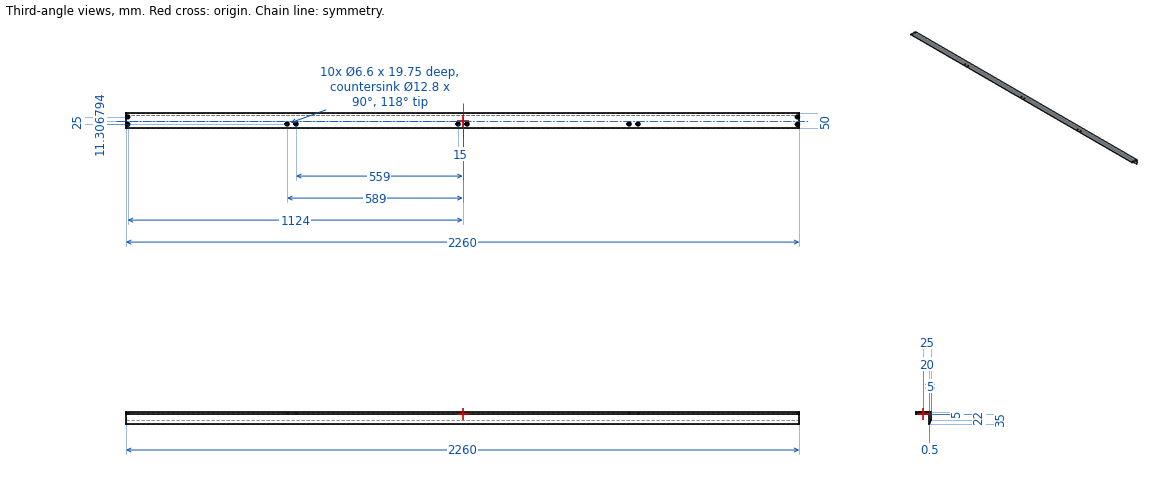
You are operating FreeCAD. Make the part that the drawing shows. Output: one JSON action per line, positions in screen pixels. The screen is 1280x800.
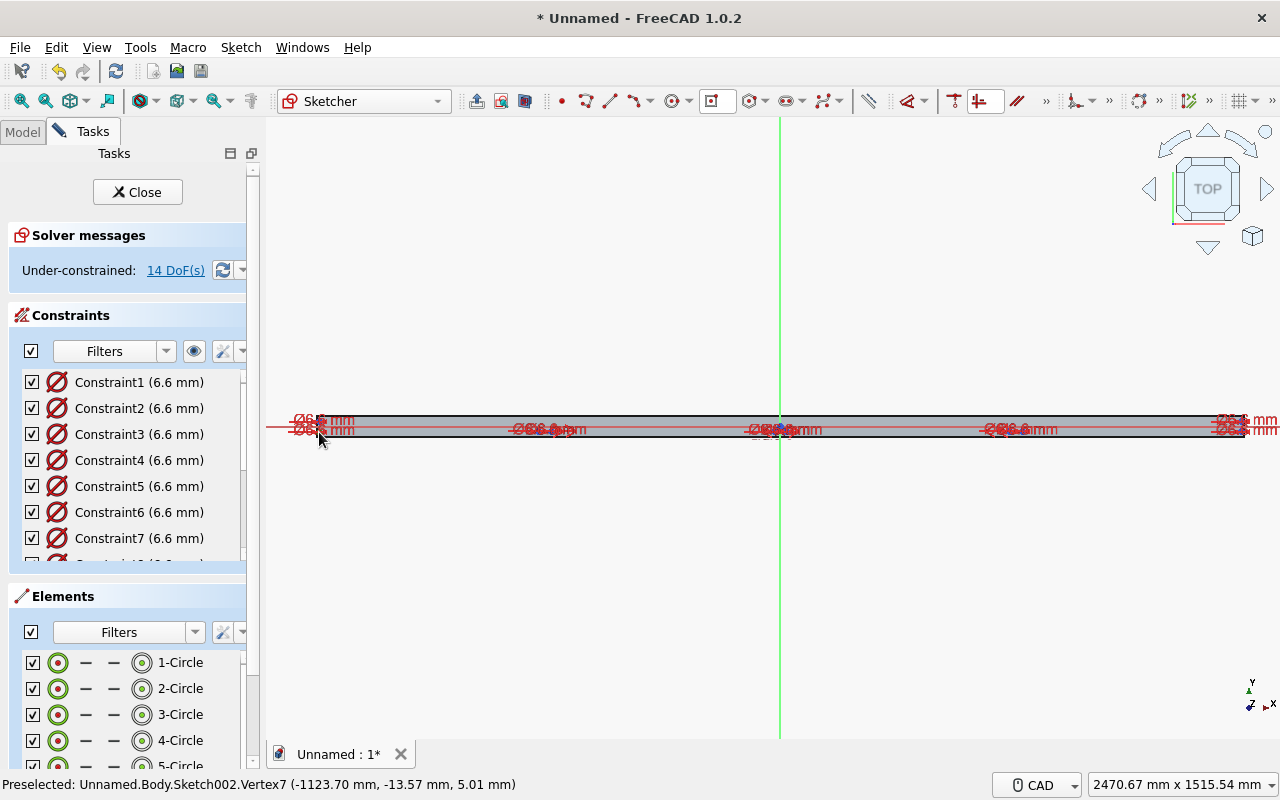
{"action": "left_click", "coordinate": [319, 422]}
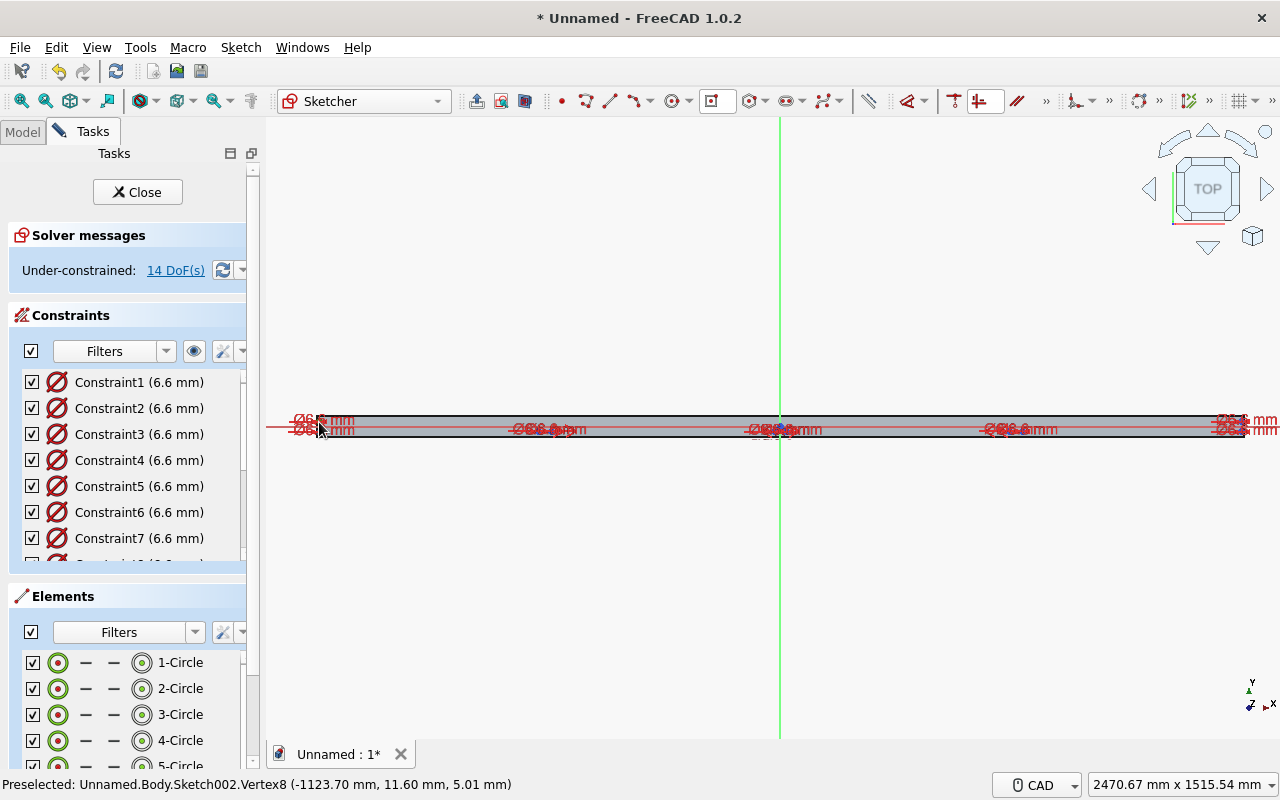
{"action": "left_click", "coordinate": [411, 427]}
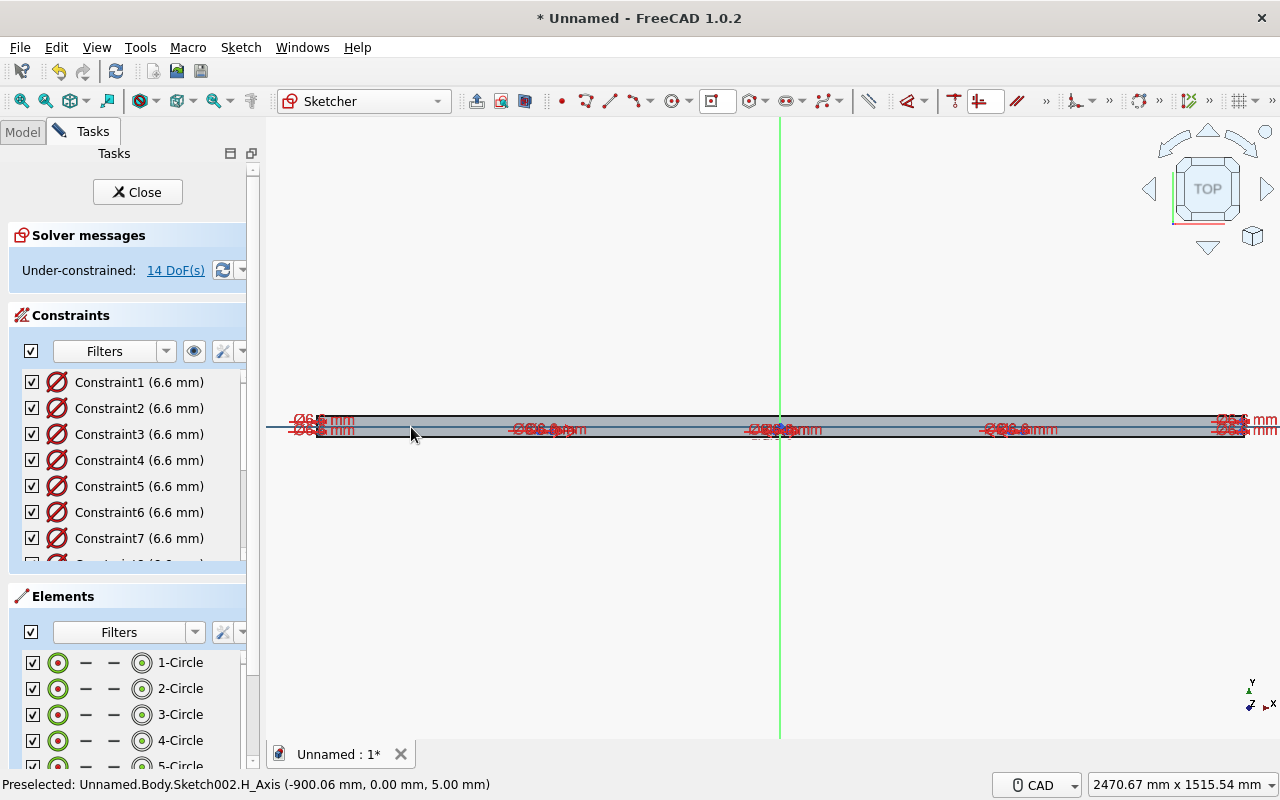
{"action": "key", "text": "s"}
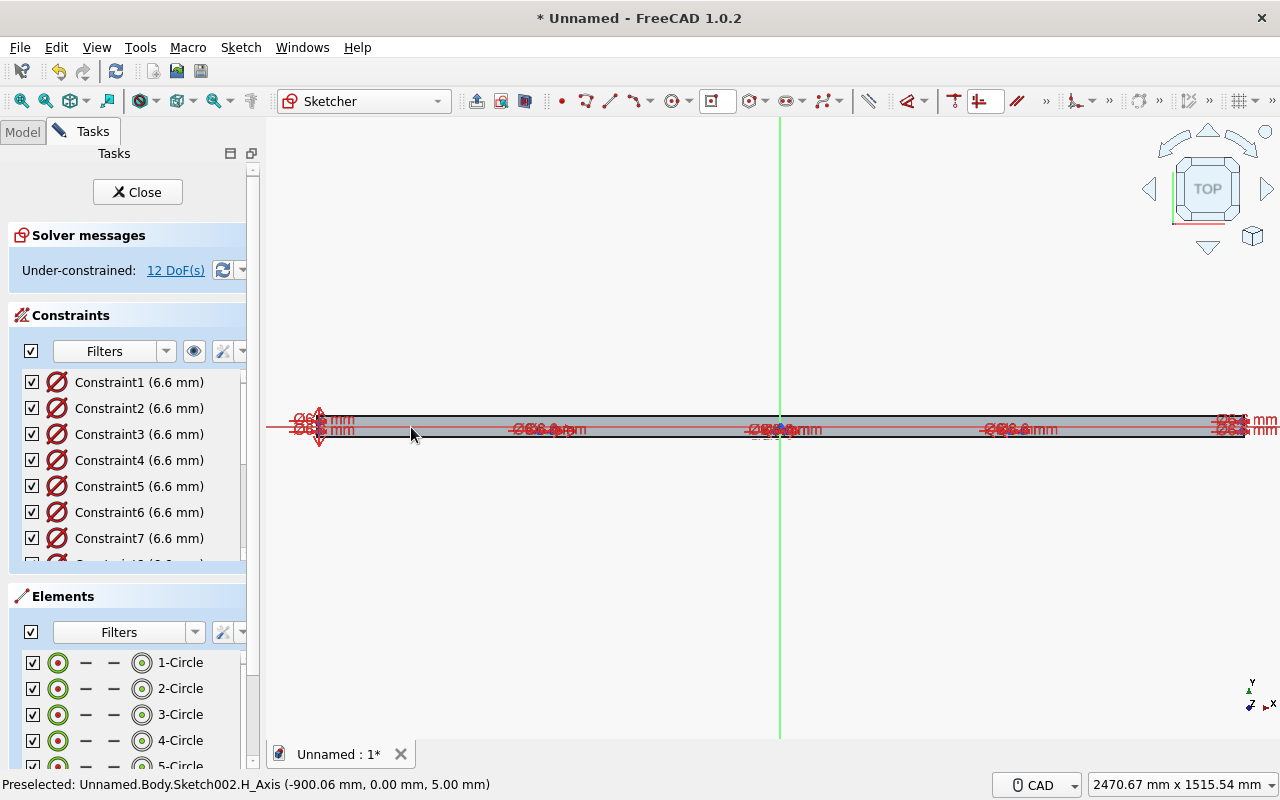
{"action": "left_click", "coordinate": [319, 432]}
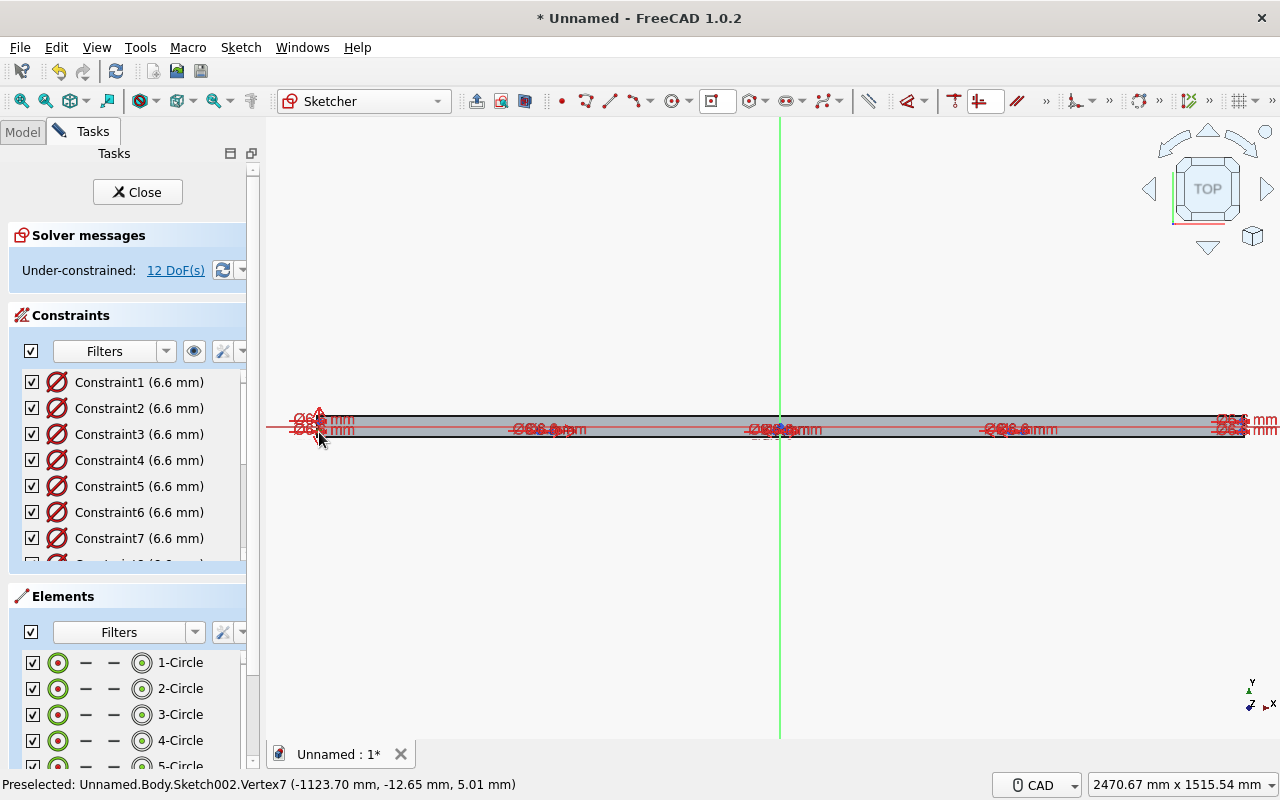
{"action": "scroll", "coordinate": [550, 431], "scroll_direction": "down", "scroll_amount": 2}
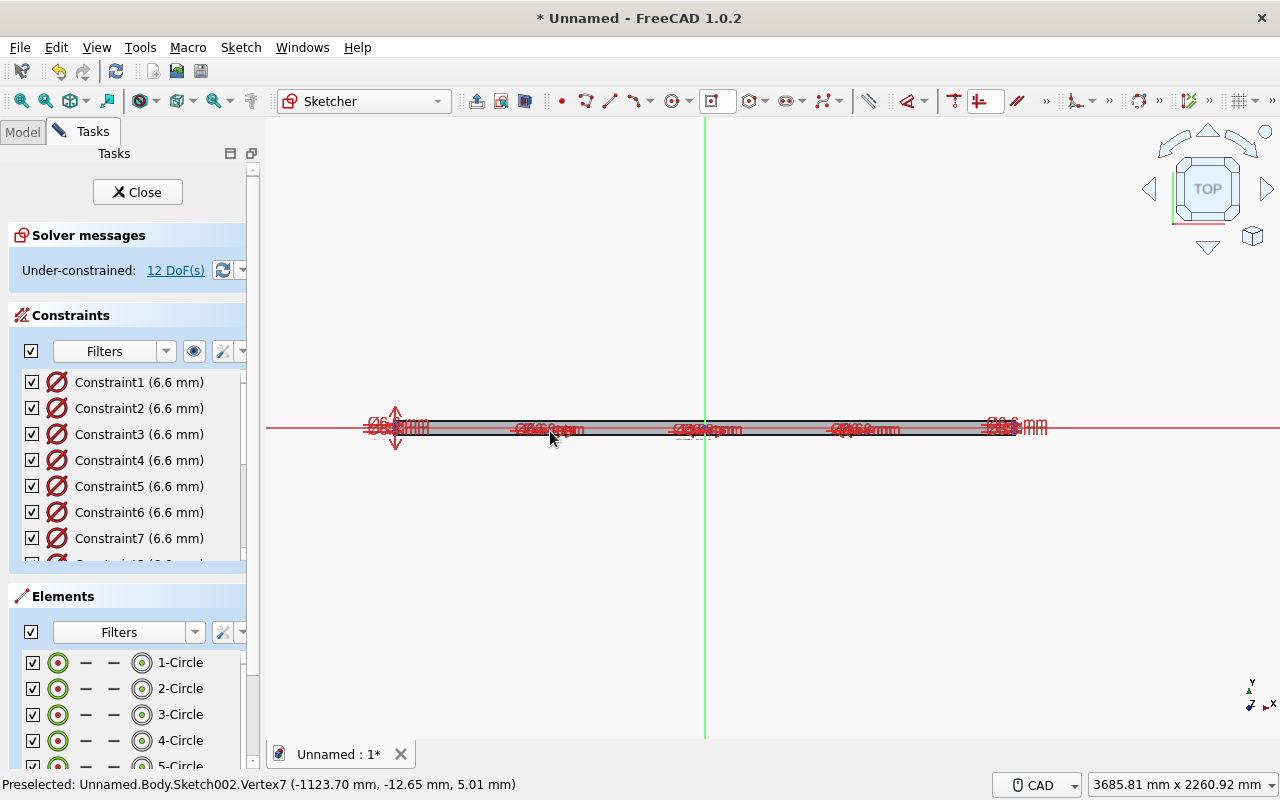
{"action": "scroll", "coordinate": [1014, 432], "scroll_direction": "up", "scroll_amount": 3}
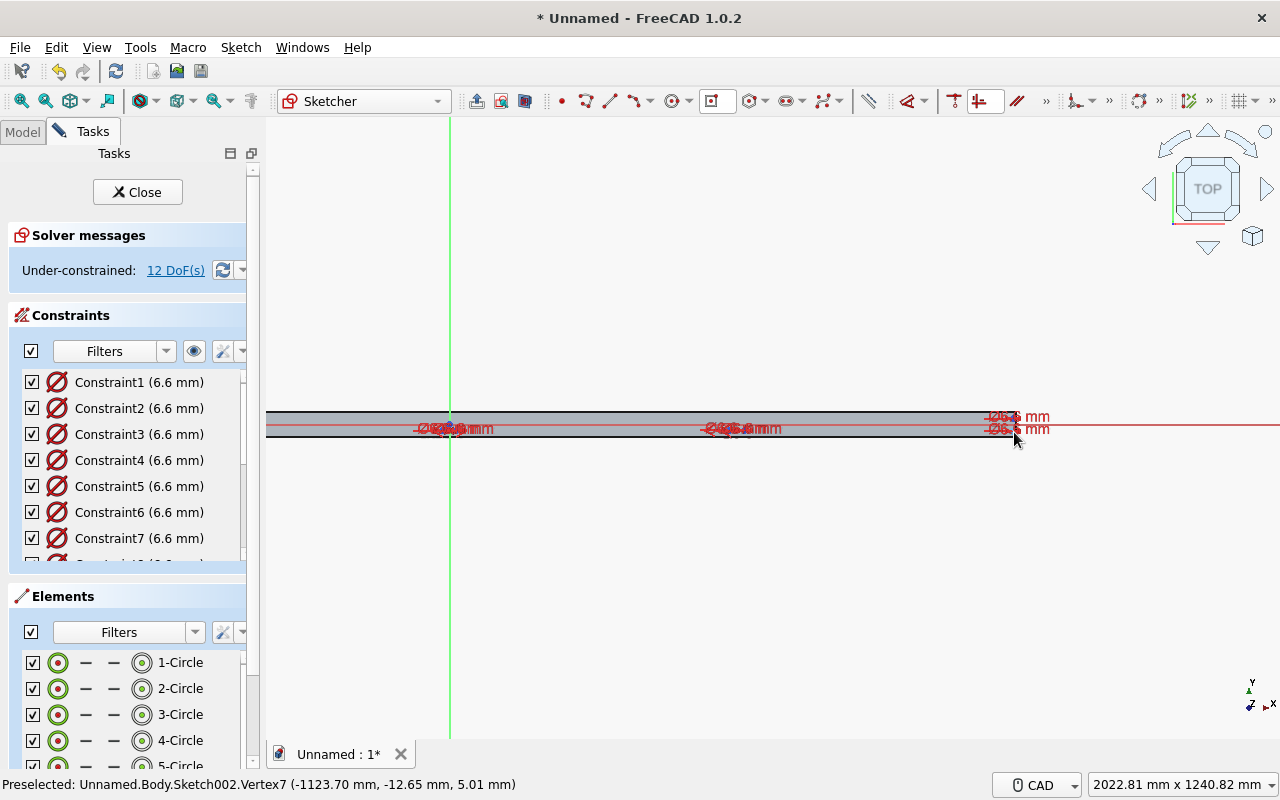
{"action": "left_click", "coordinate": [1013, 431]}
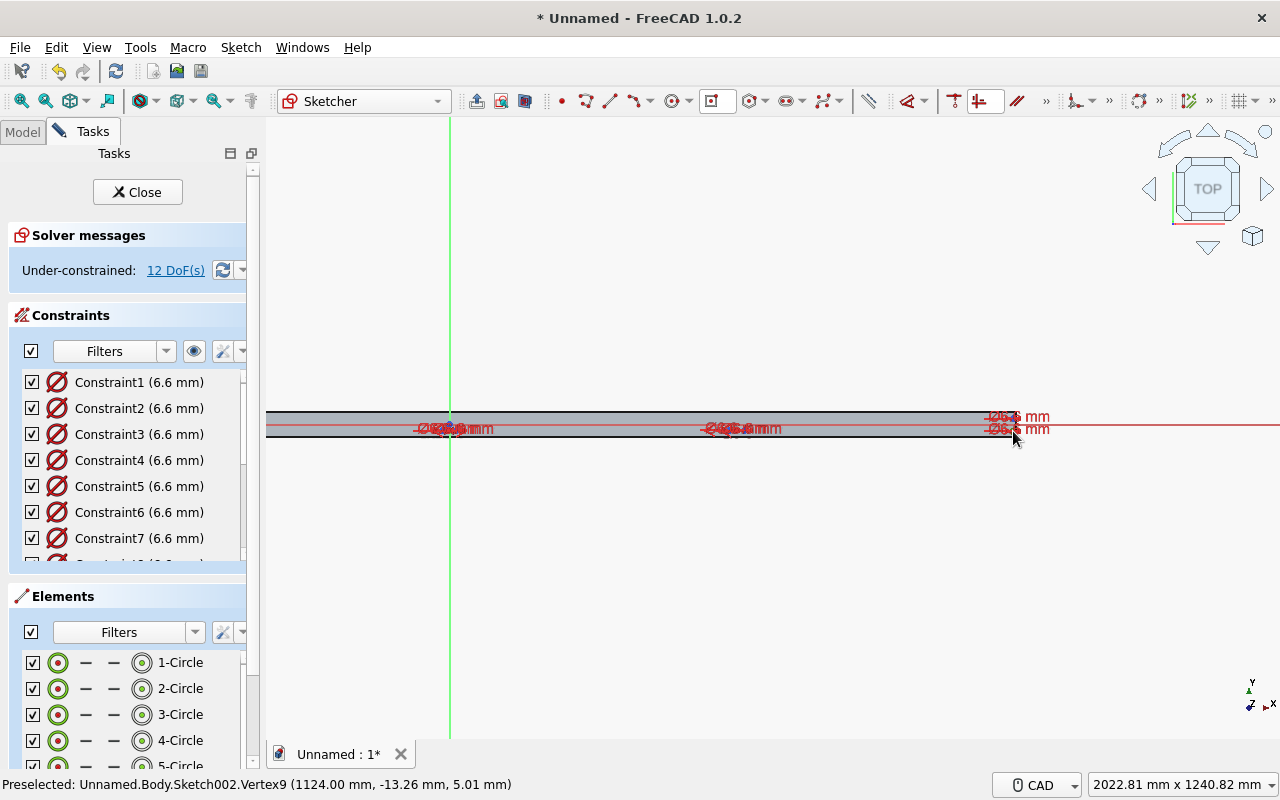
{"action": "left_click", "coordinate": [450, 671]}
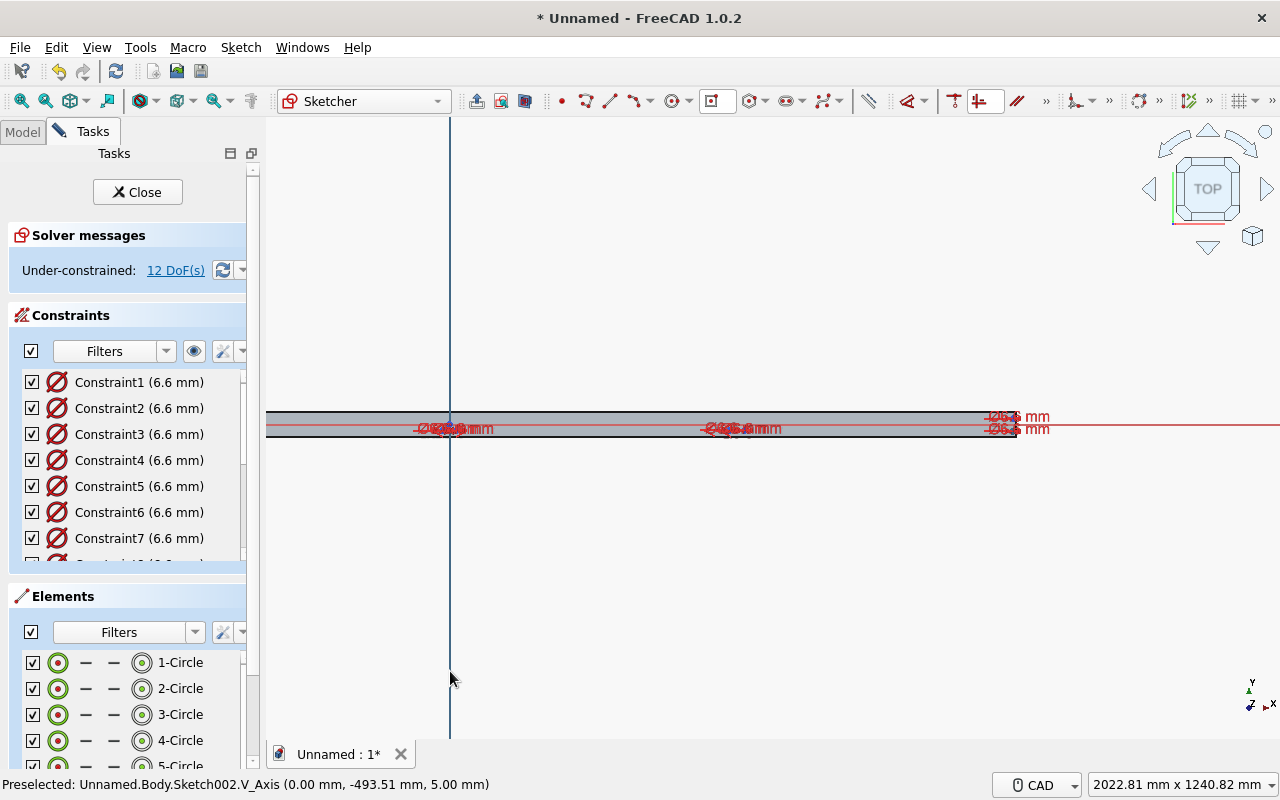
{"action": "key", "text": "s"}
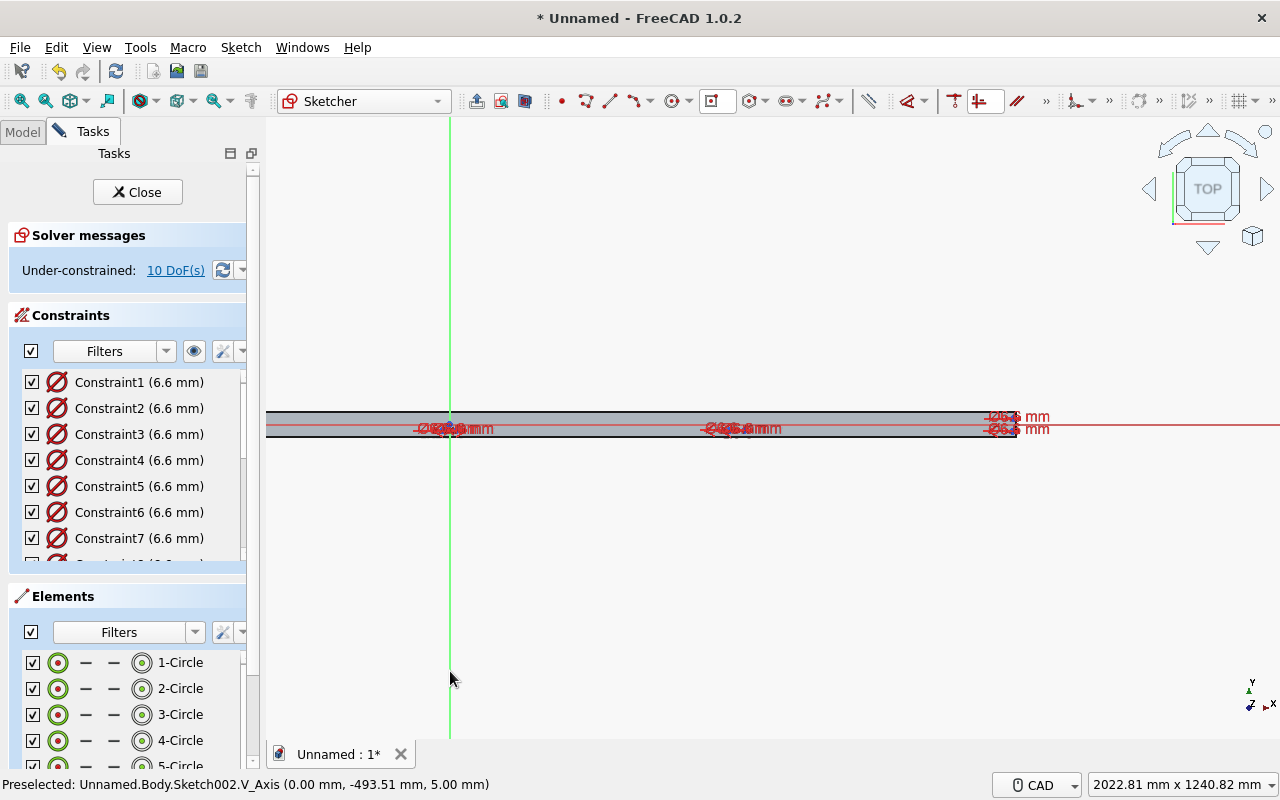
{"action": "scroll", "coordinate": [1015, 432], "scroll_direction": "down", "scroll_amount": 3}